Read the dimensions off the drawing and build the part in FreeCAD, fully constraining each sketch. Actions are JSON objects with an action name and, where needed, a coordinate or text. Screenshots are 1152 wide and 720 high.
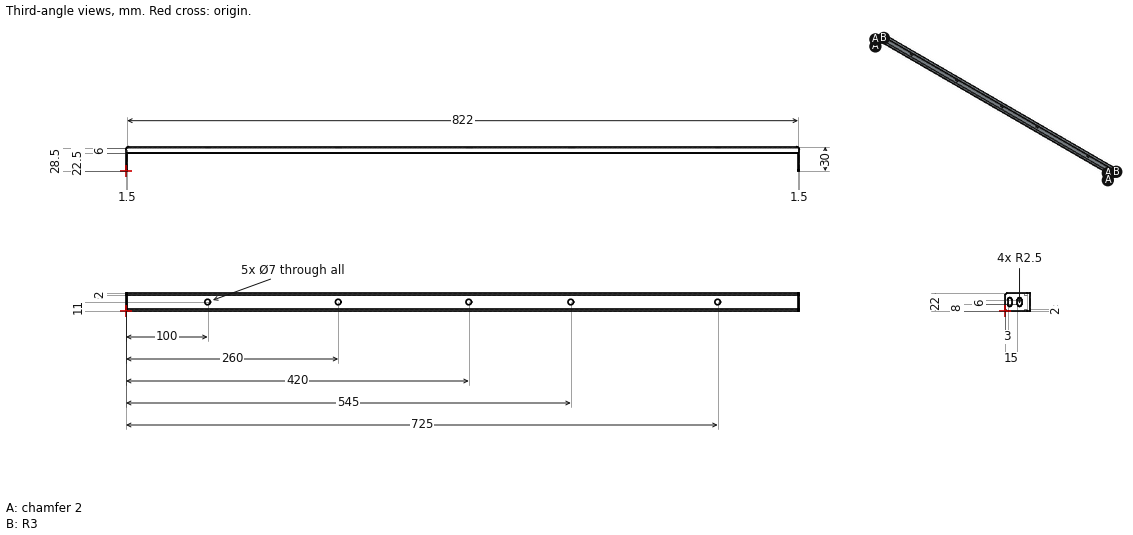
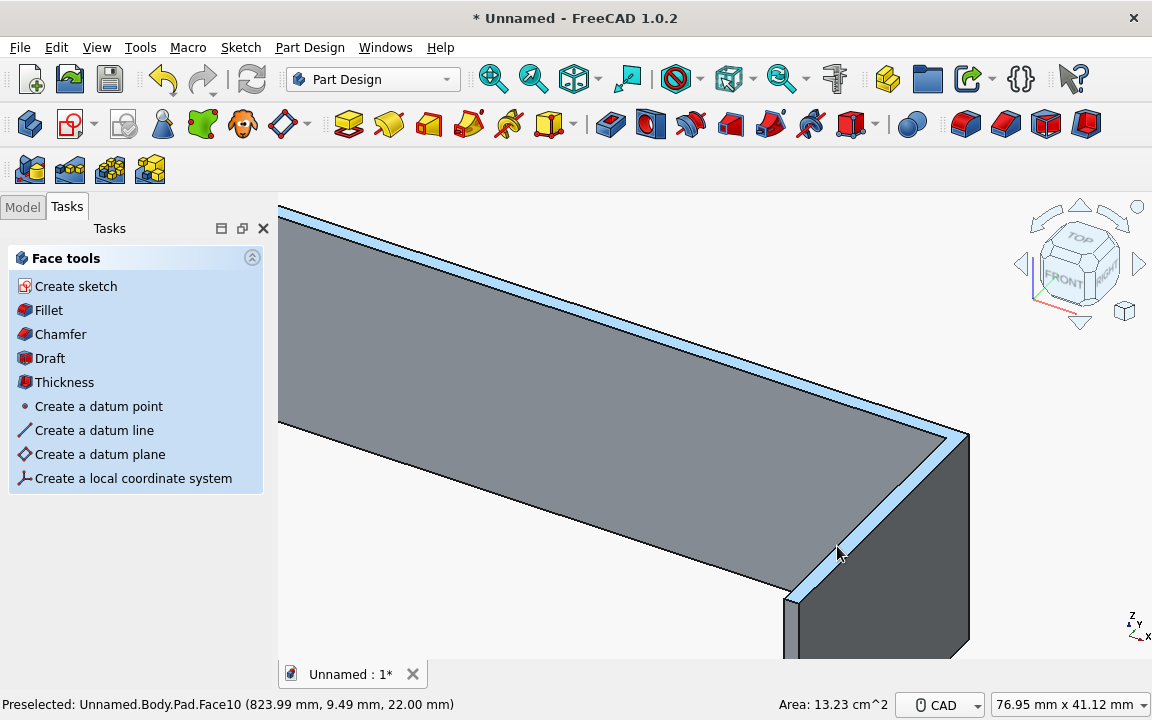
{"action": "left_click", "coordinate": [70, 124]}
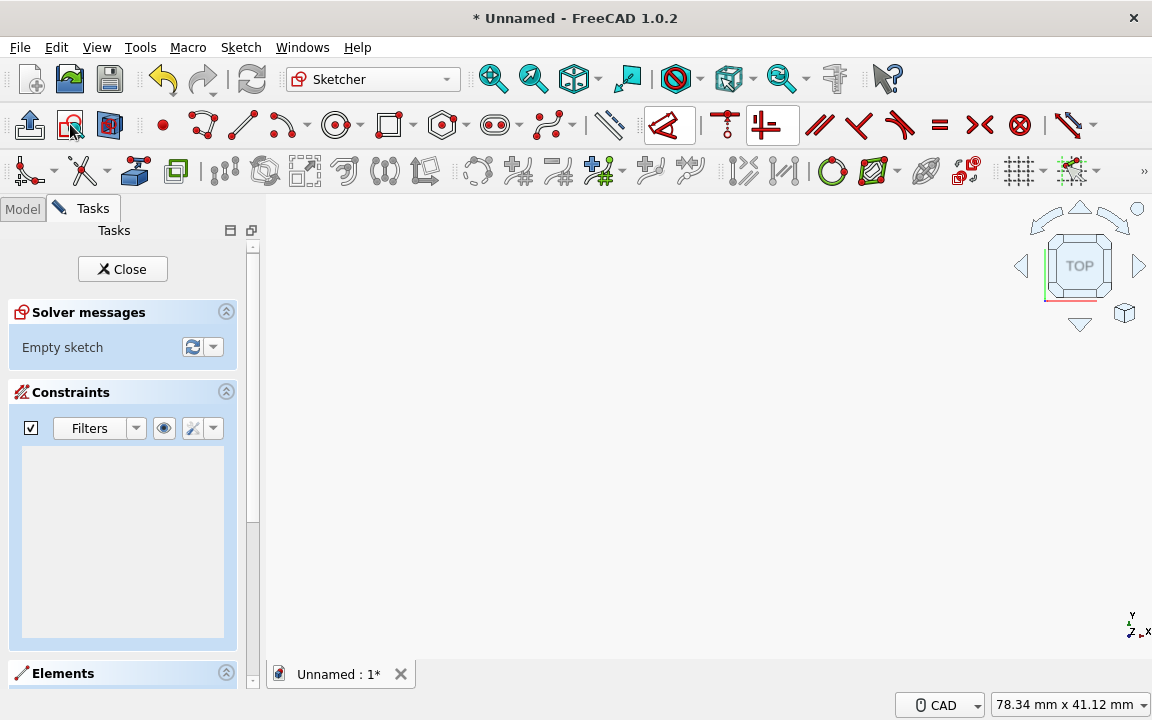
{"action": "scroll", "coordinate": [830, 354], "scroll_direction": "down", "scroll_amount": 15}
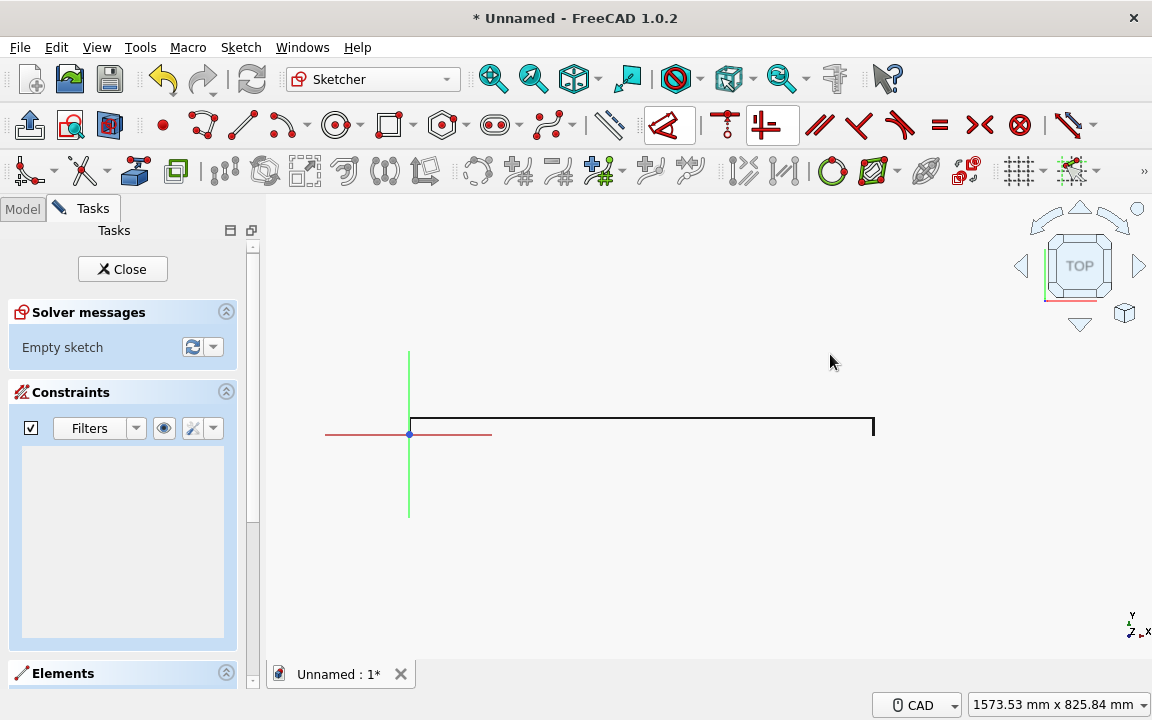
{"action": "left_click", "coordinate": [390, 126]}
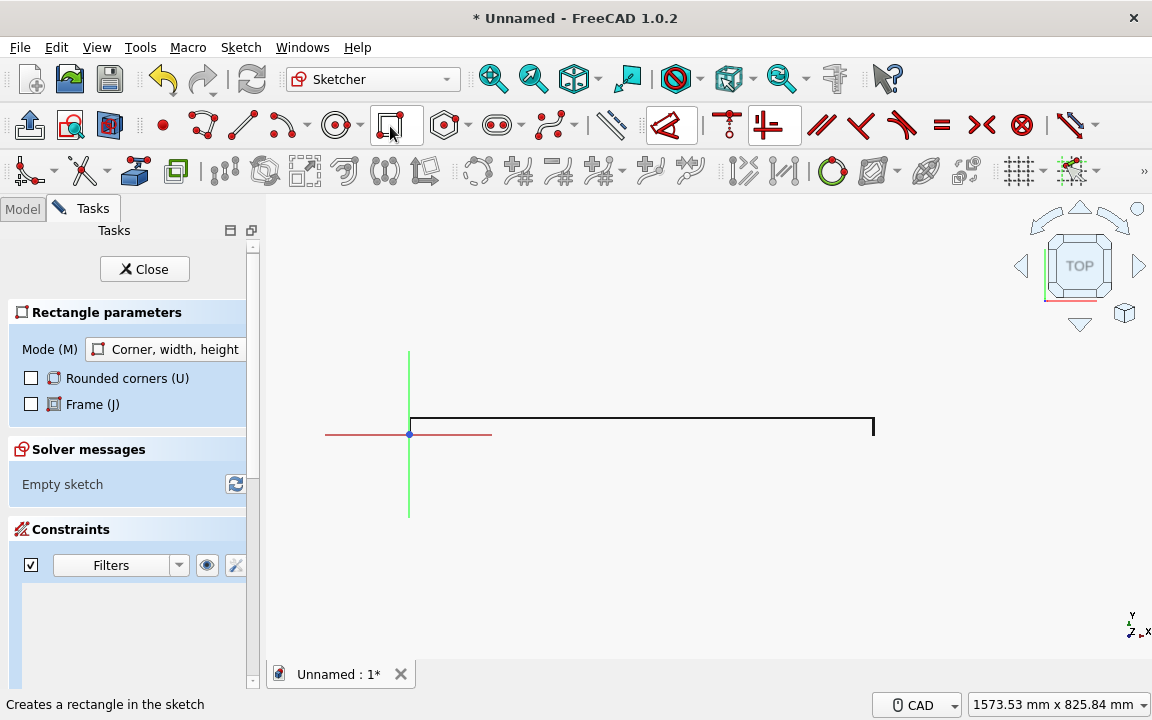
{"action": "scroll", "coordinate": [410, 418], "scroll_direction": "up", "scroll_amount": 15}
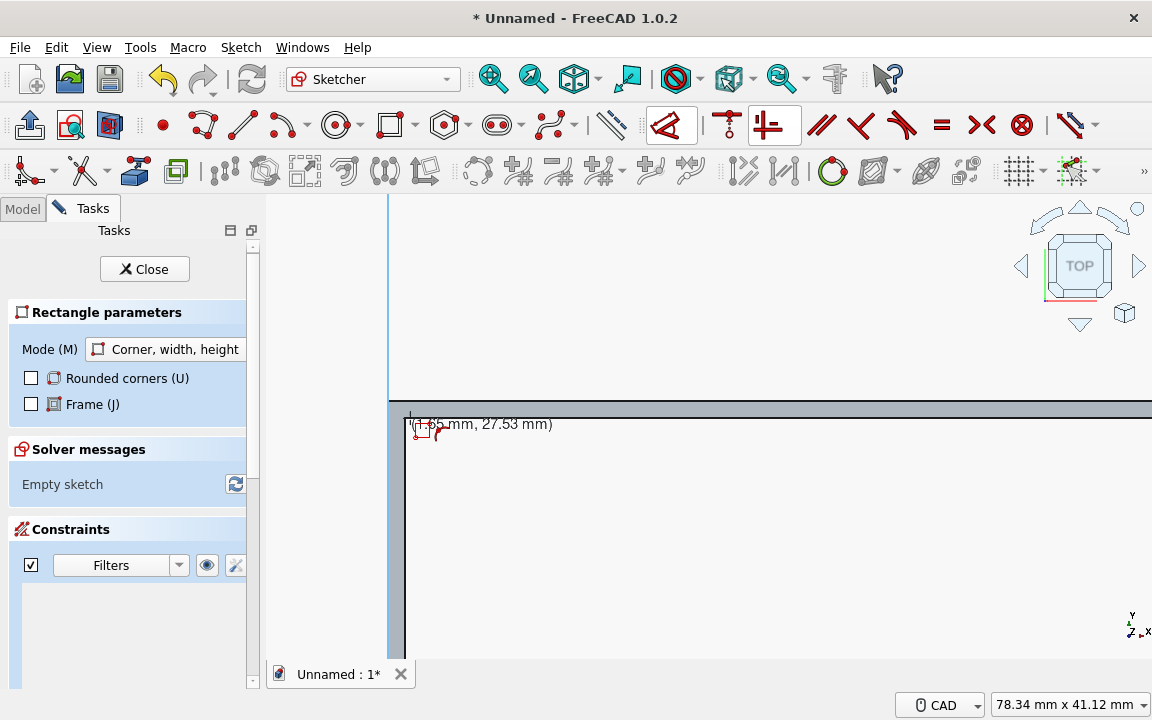
{"action": "left_click", "coordinate": [405, 418]}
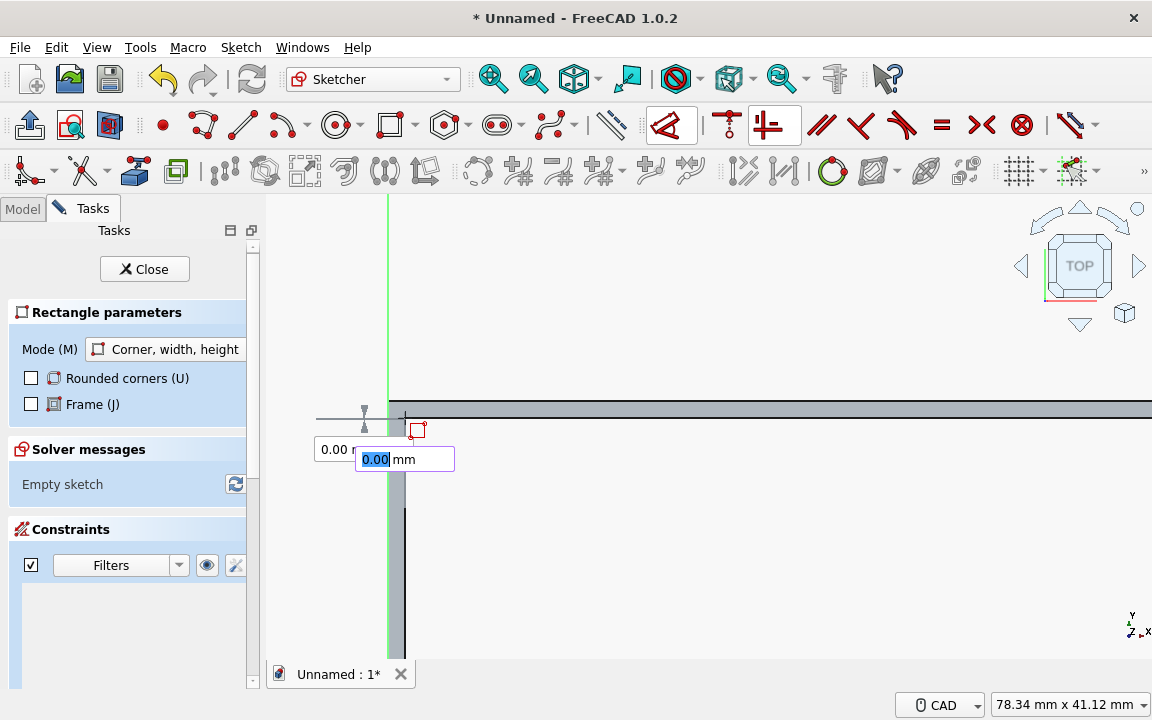
{"action": "scroll", "coordinate": [410, 419], "scroll_direction": "down", "scroll_amount": 15}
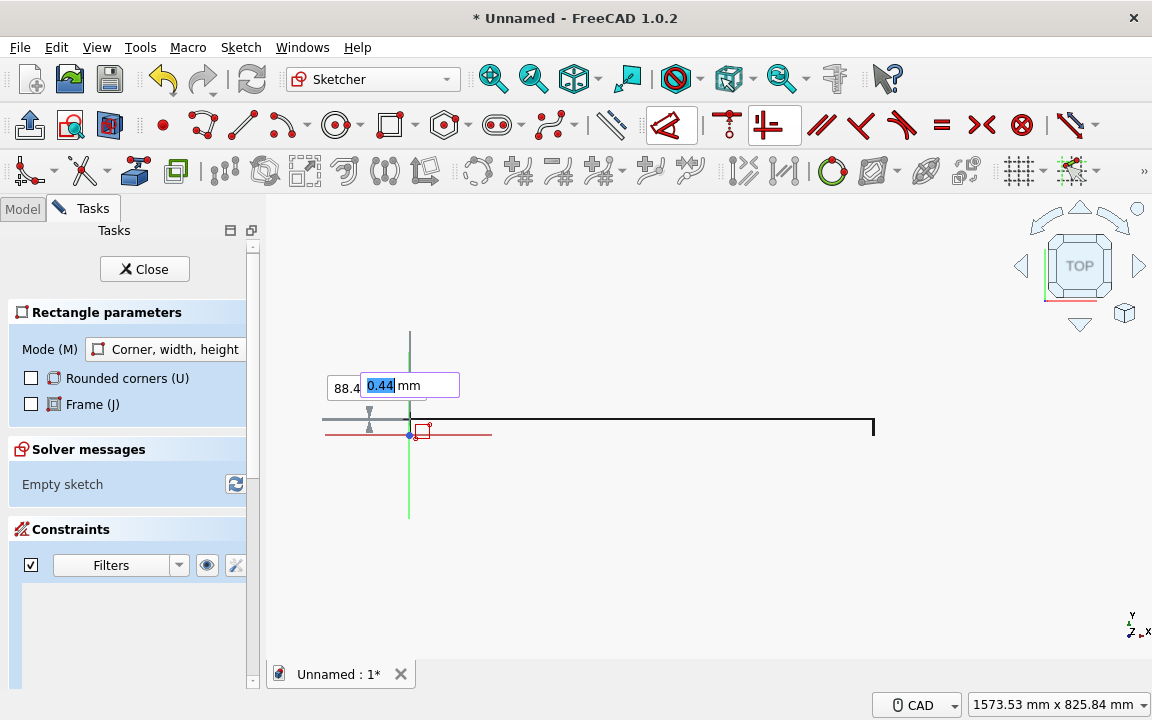
{"action": "scroll", "coordinate": [873, 423], "scroll_direction": "up", "scroll_amount": 2}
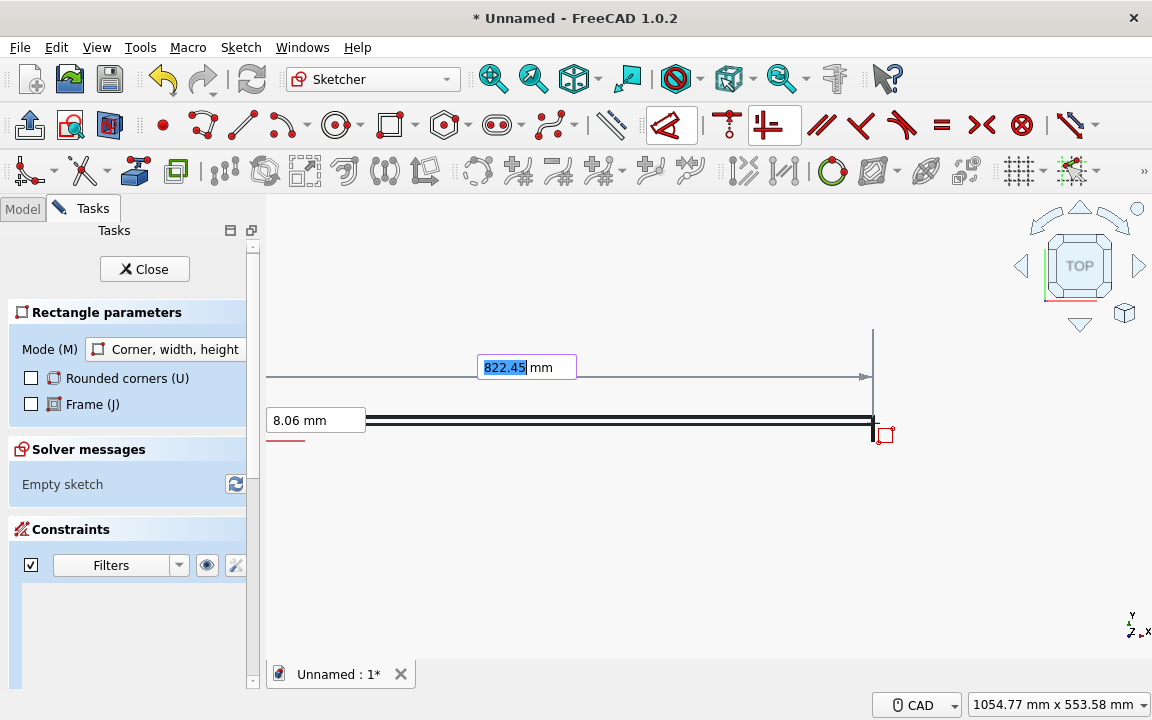
{"action": "left_click", "coordinate": [872, 422]}
{"action": "key", "text": "Escape"}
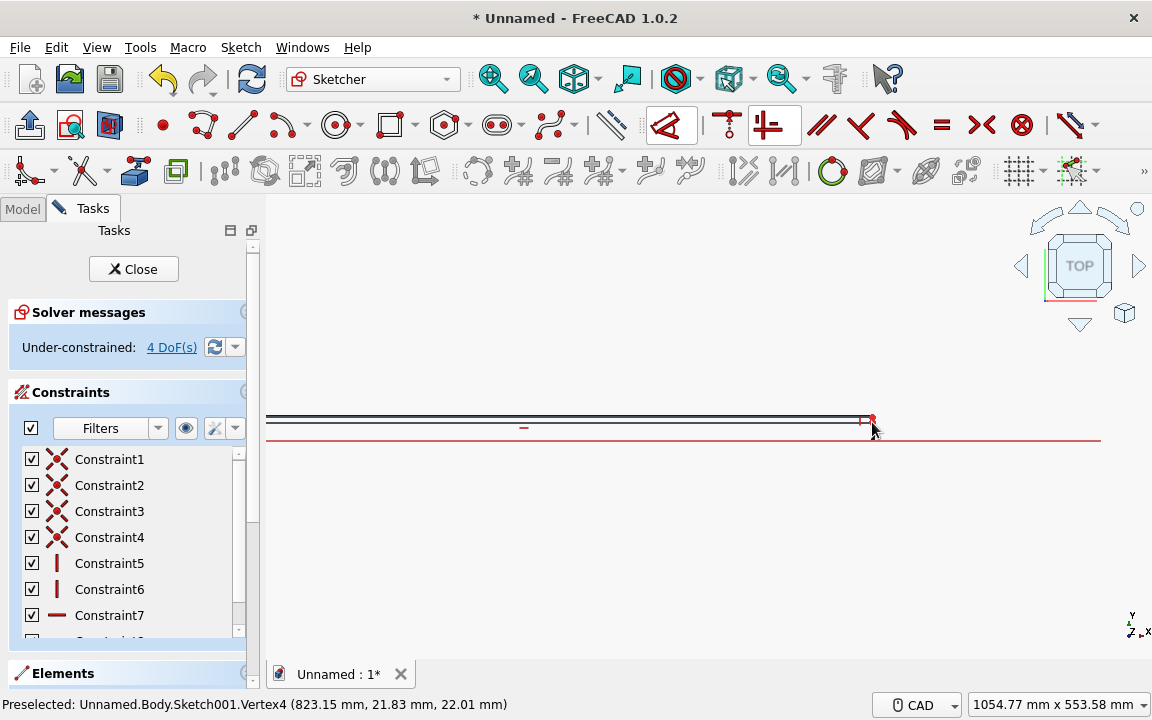
{"action": "scroll", "coordinate": [872, 421], "scroll_direction": "down", "scroll_amount": 2}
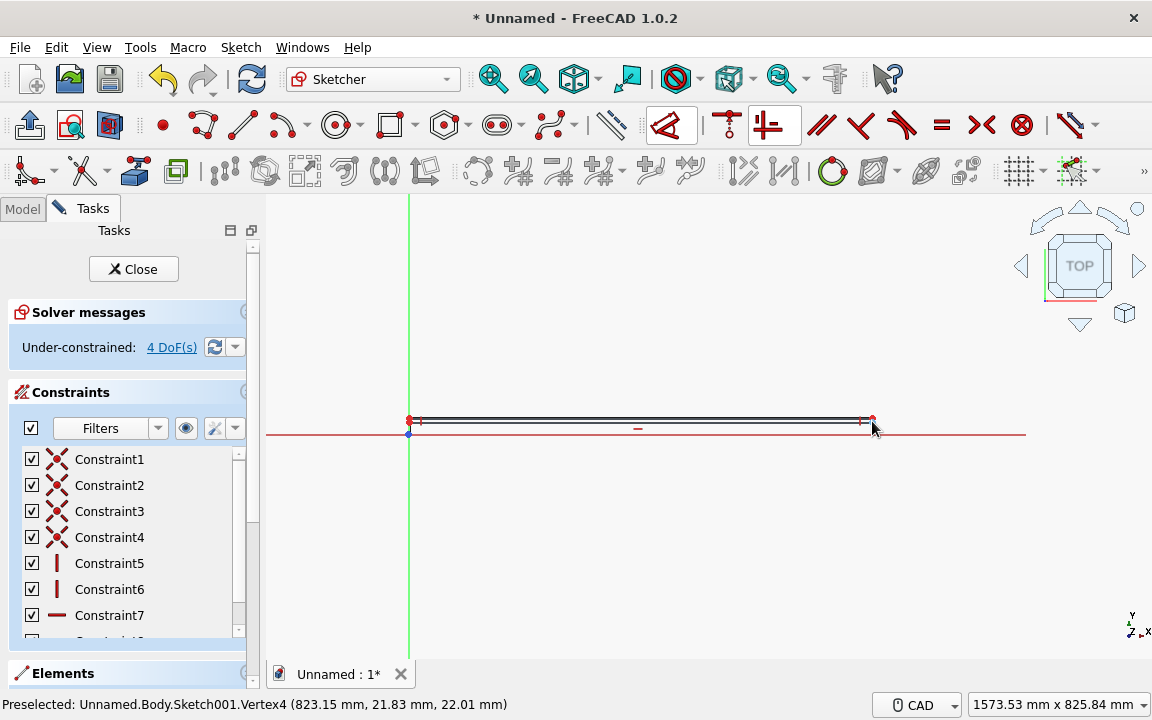
{"action": "scroll", "coordinate": [410, 421], "scroll_direction": "up", "scroll_amount": 13}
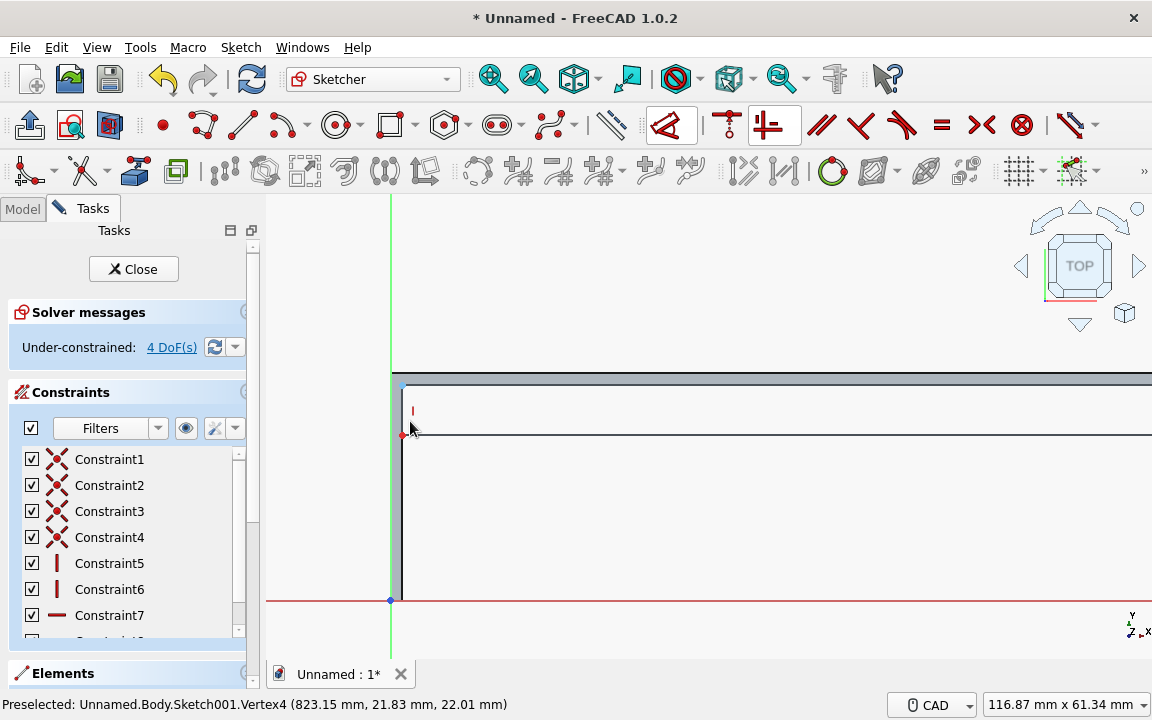
{"action": "left_click", "coordinate": [402, 410]}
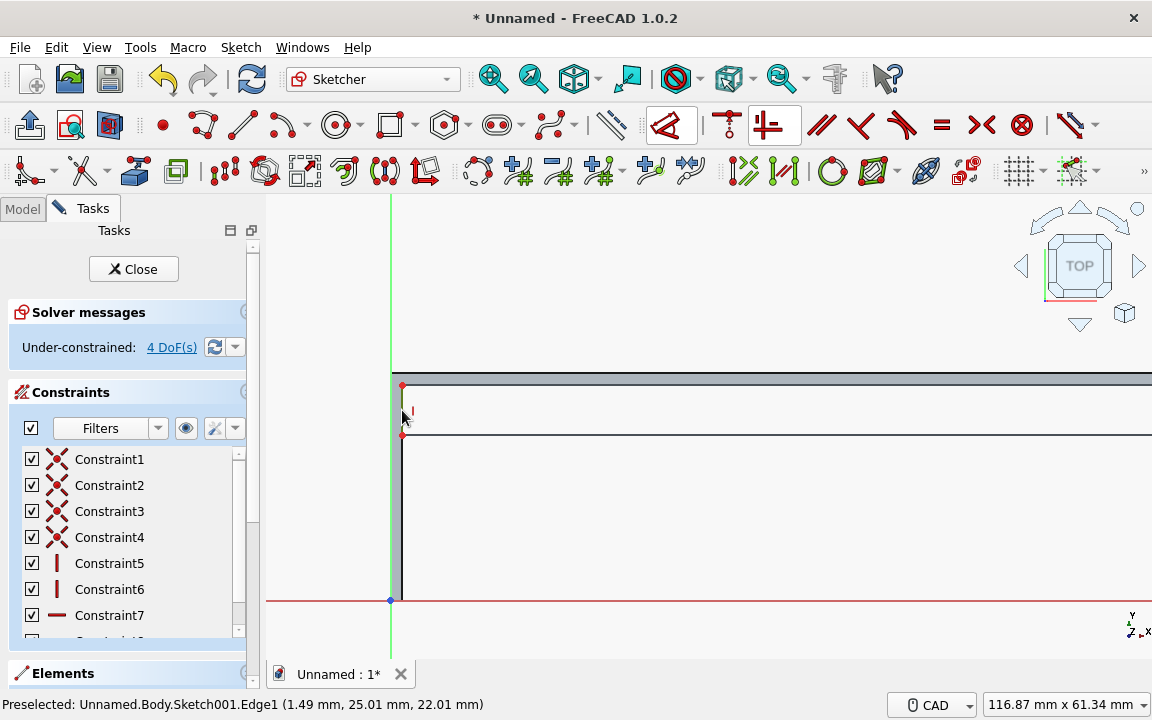
{"action": "key", "text": "i"}